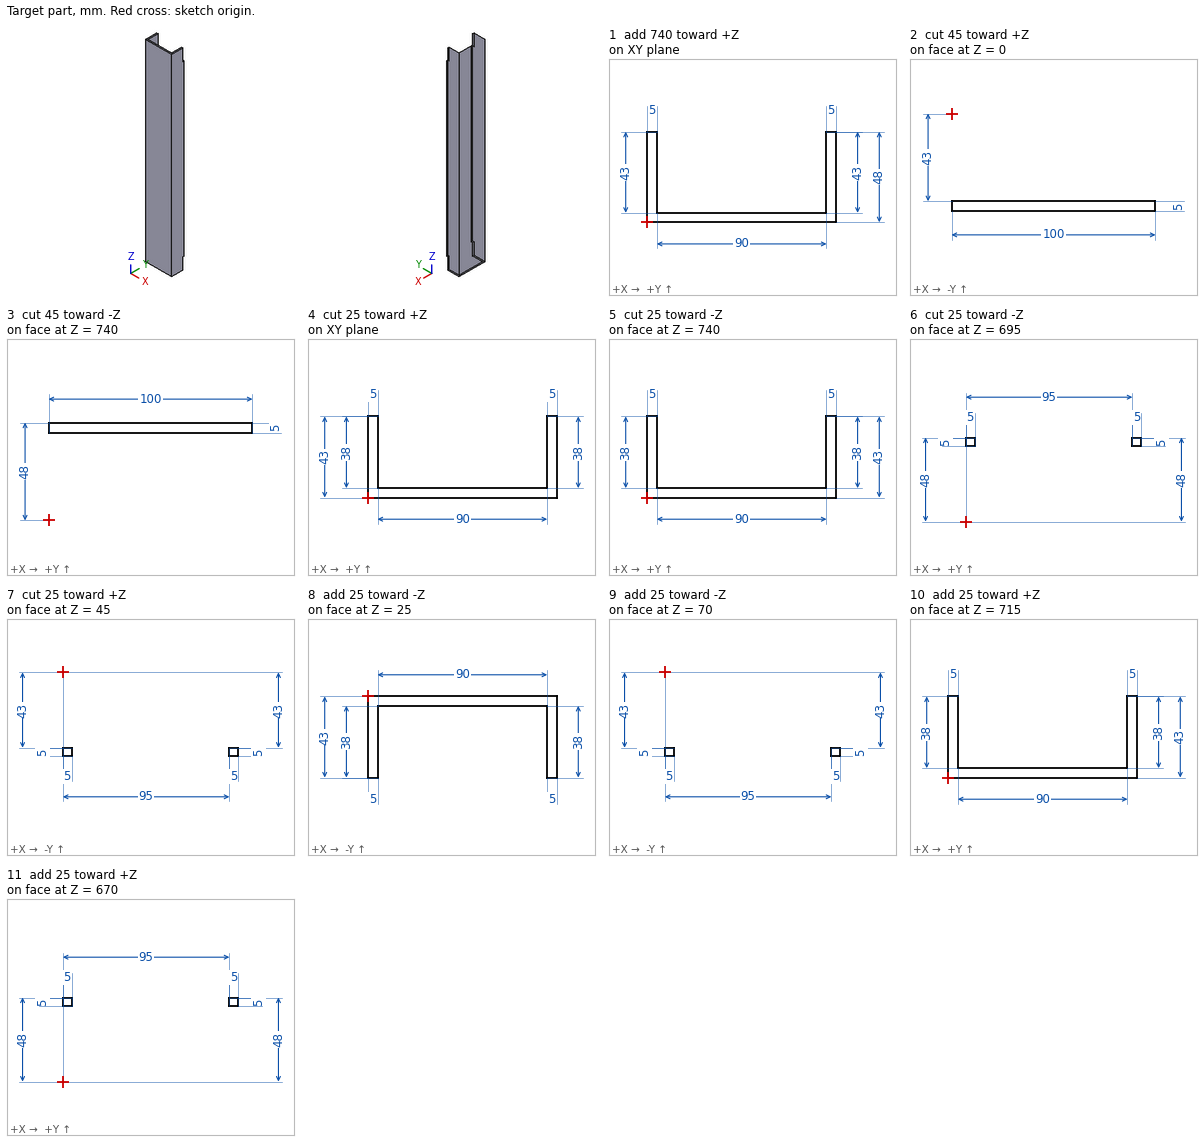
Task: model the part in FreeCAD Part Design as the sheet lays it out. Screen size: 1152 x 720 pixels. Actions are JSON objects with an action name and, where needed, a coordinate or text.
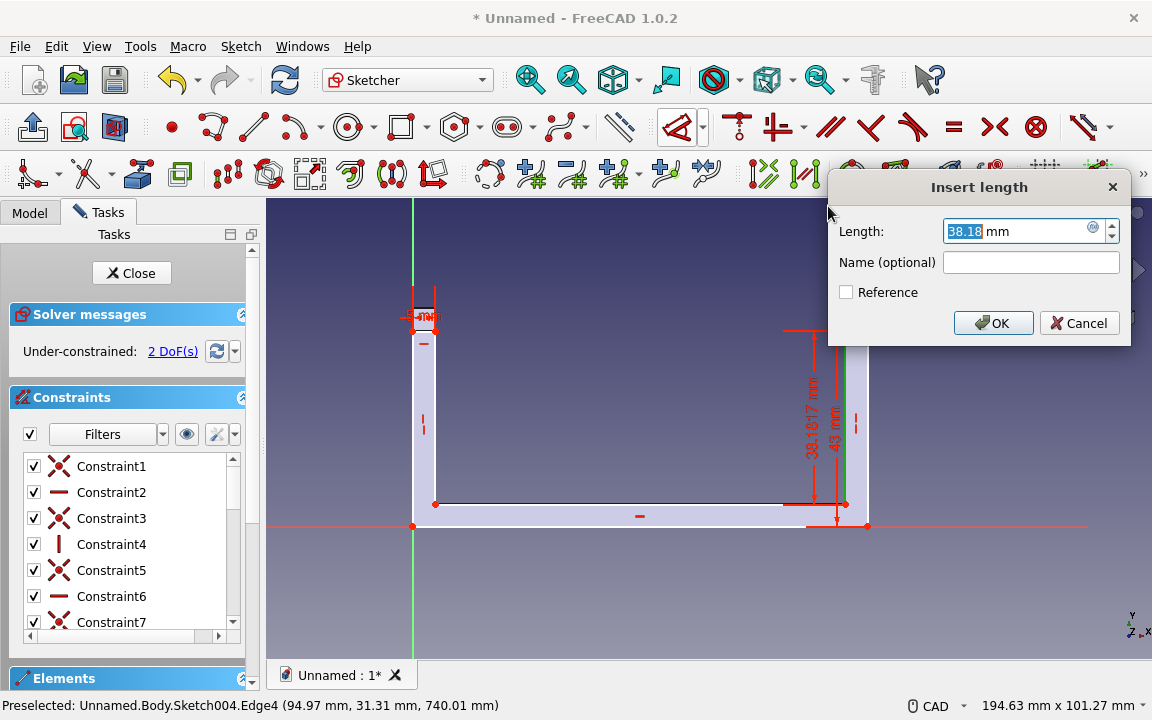
{"action": "type", "text": "38"}
{"action": "key", "text": "Return"}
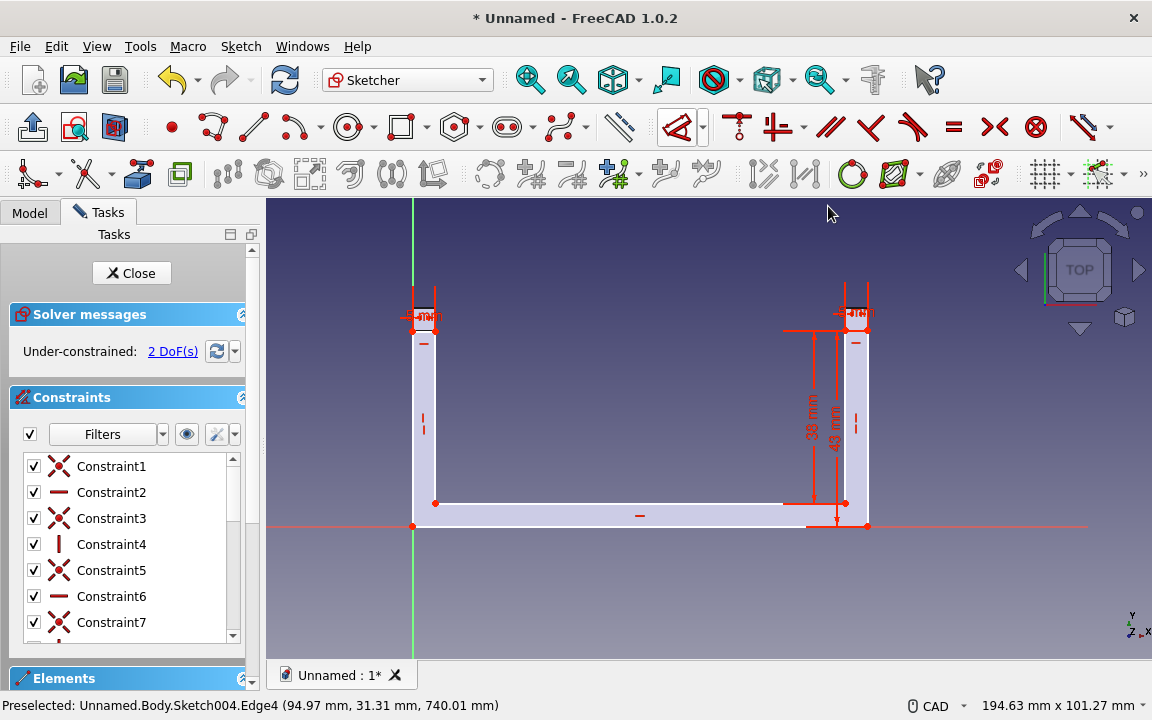
{"action": "left_click", "coordinate": [722, 504]}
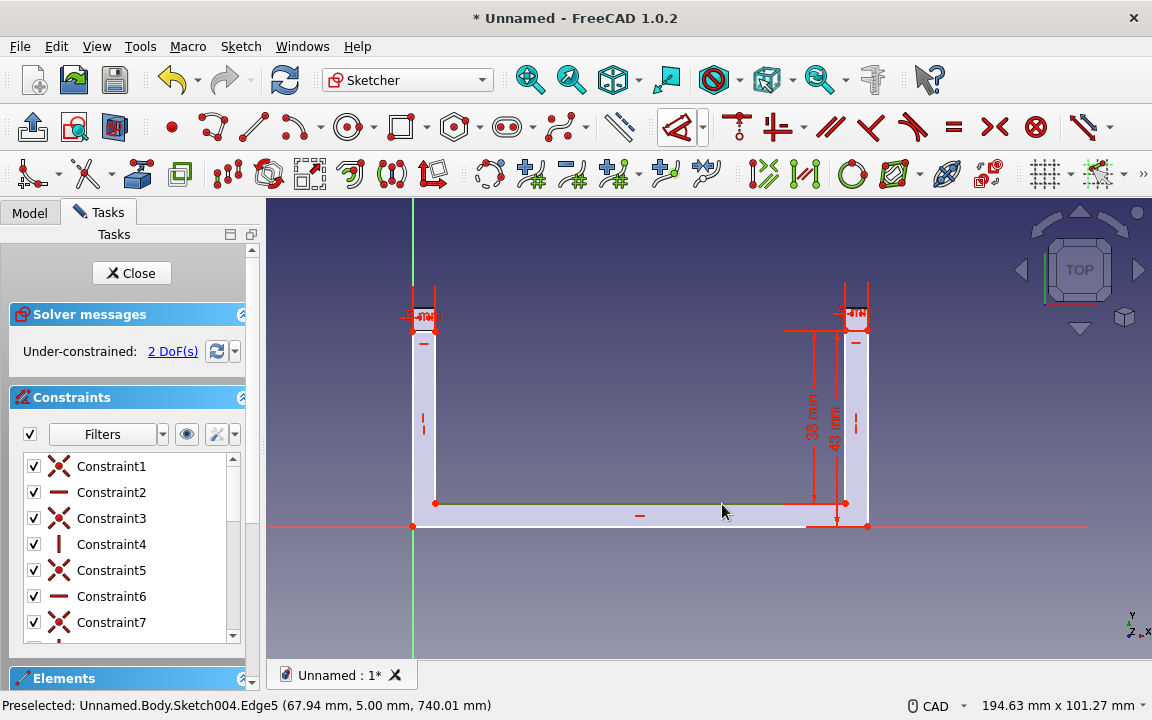
{"action": "key", "text": "l"}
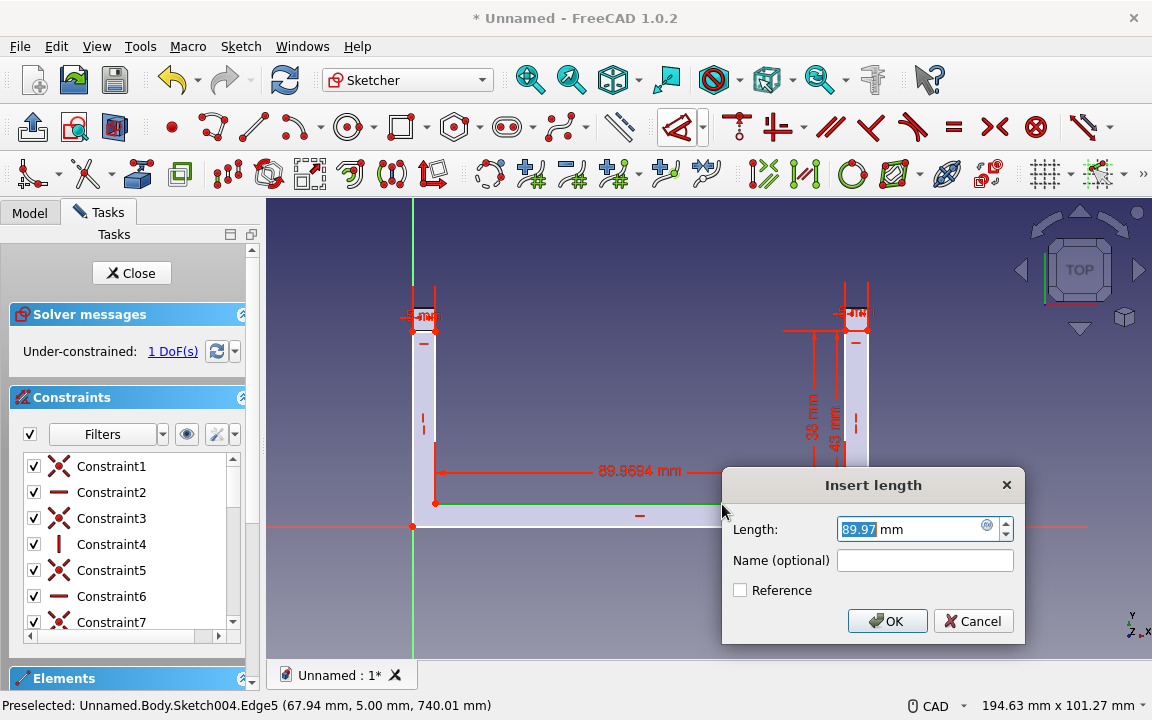
{"action": "type", "text": "90"}
{"action": "key", "text": "Return"}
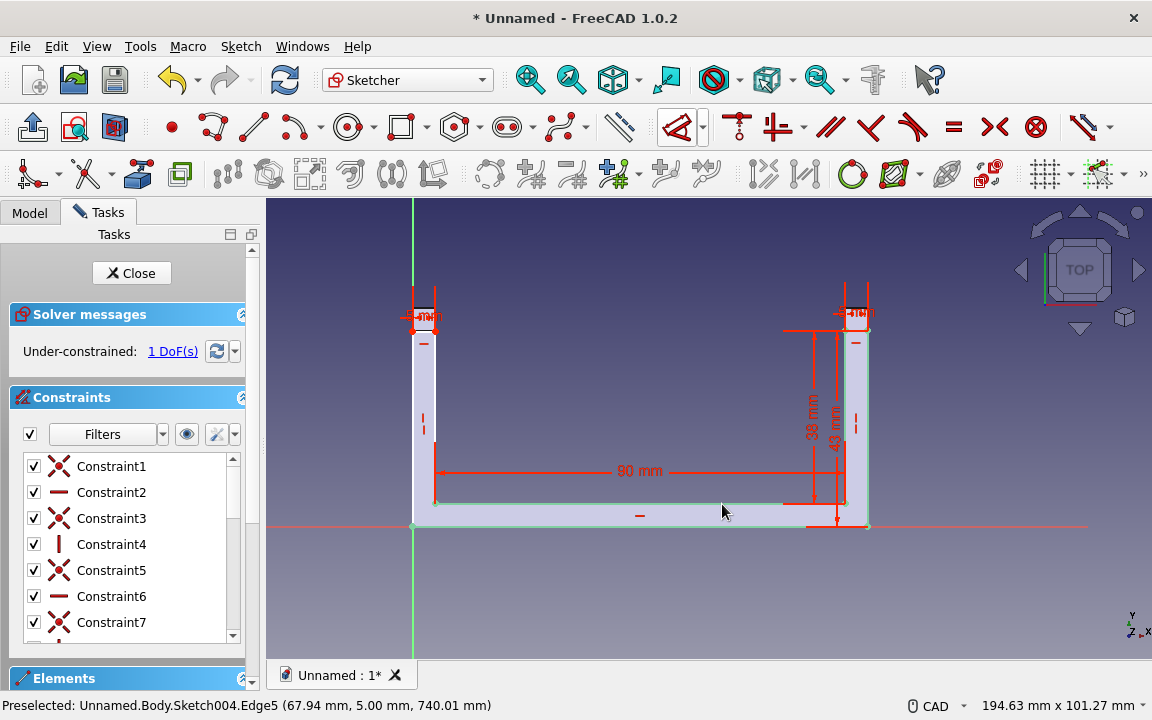
{"action": "left_click", "coordinate": [435, 452]}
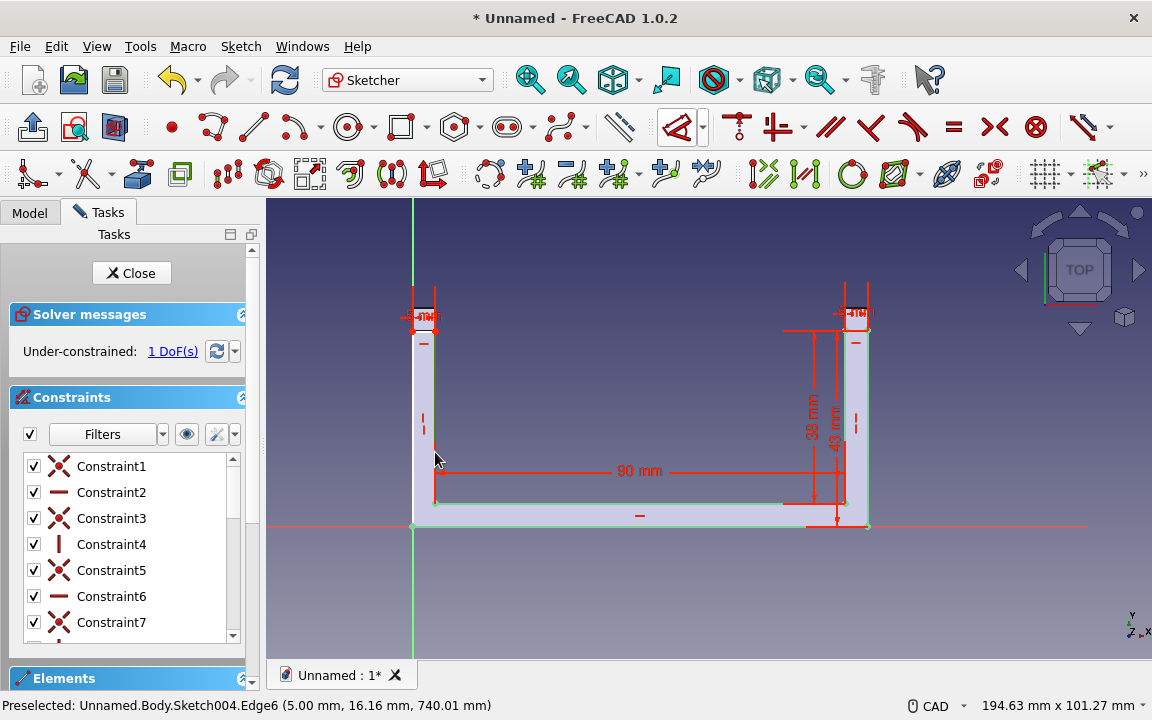
{"action": "key", "text": "i"}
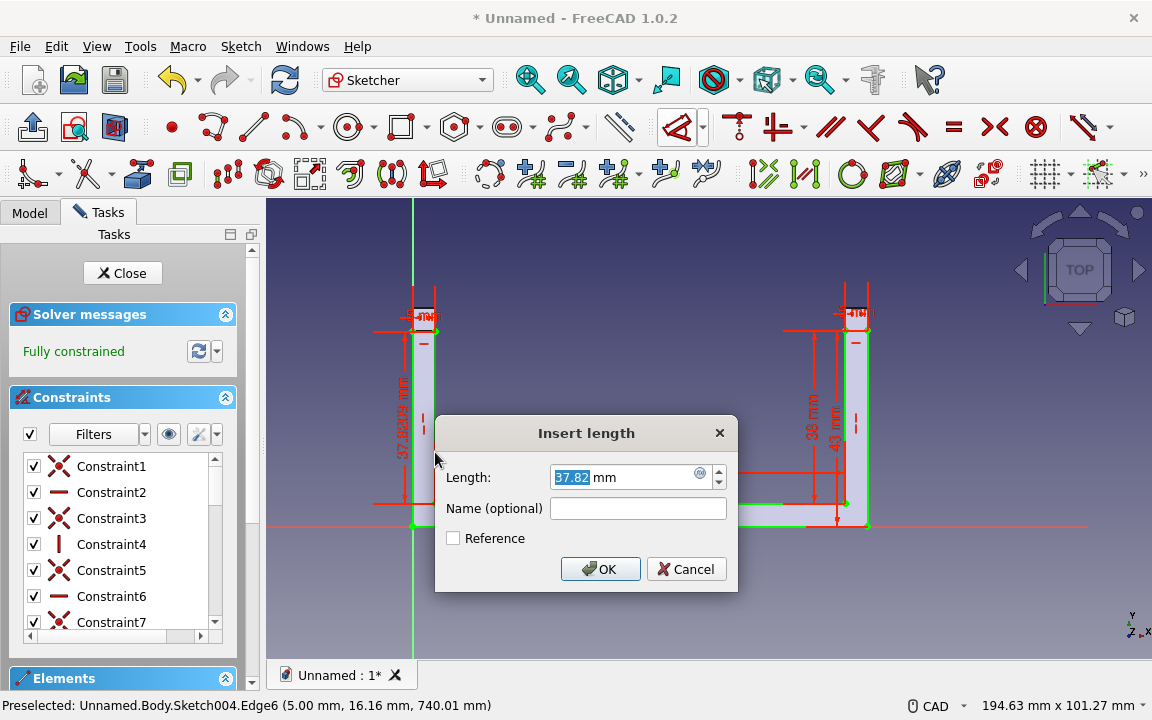
{"action": "type", "text": "38"}
{"action": "key", "text": "Return"}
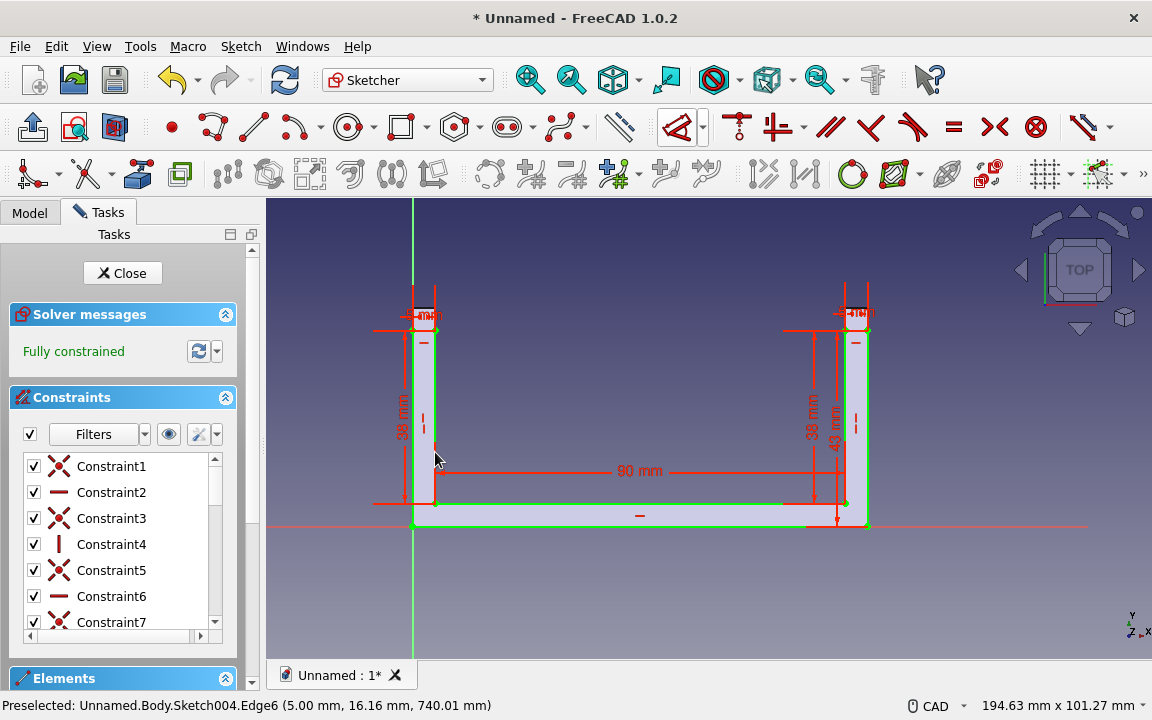
{"action": "left_click", "coordinate": [123, 273]}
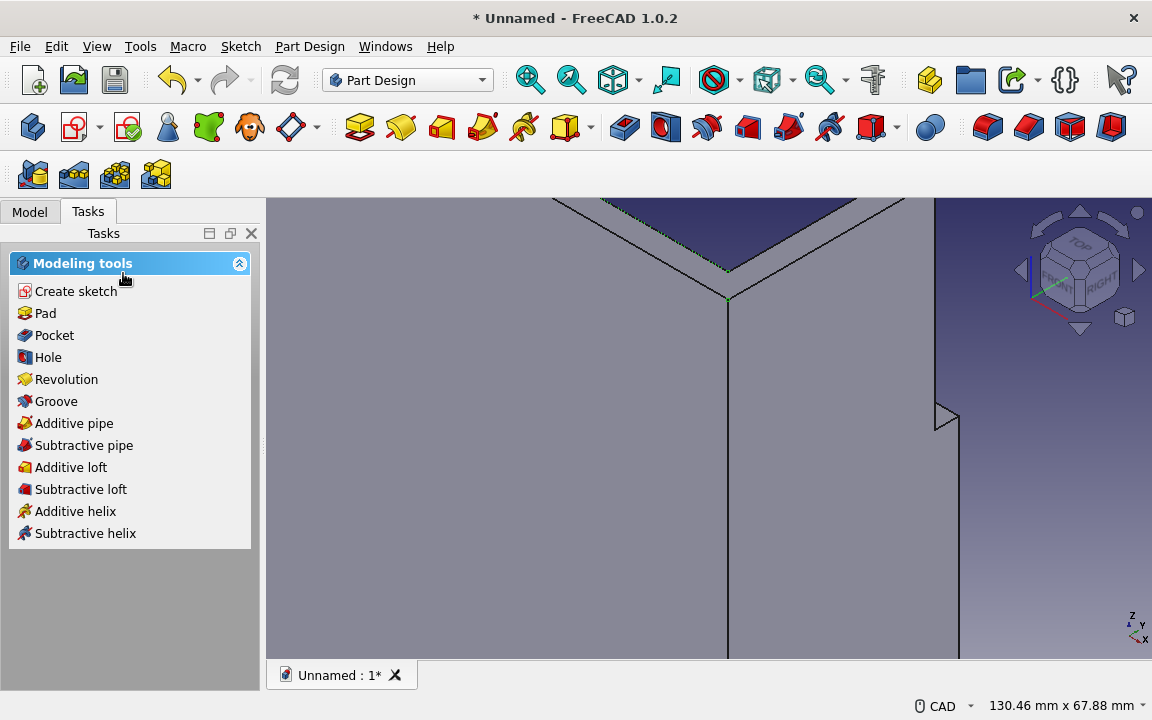
{"action": "left_click", "coordinate": [625, 128]}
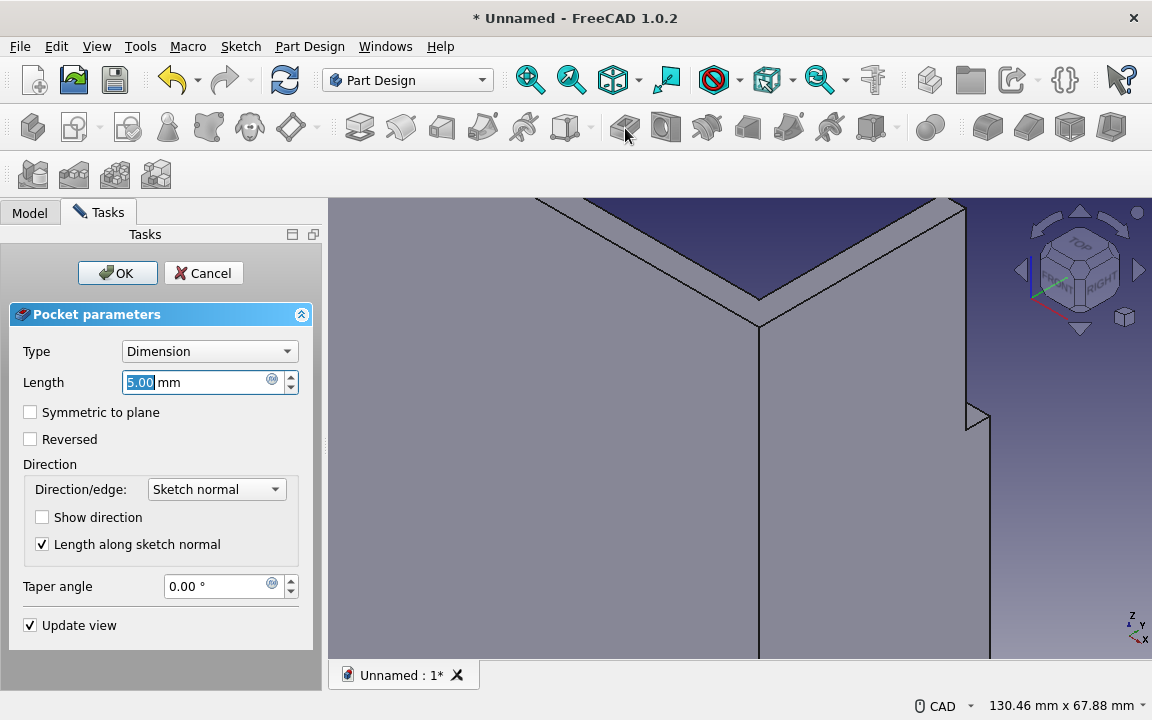
{"action": "type", "text": "25"}
{"action": "key", "text": "Tab"}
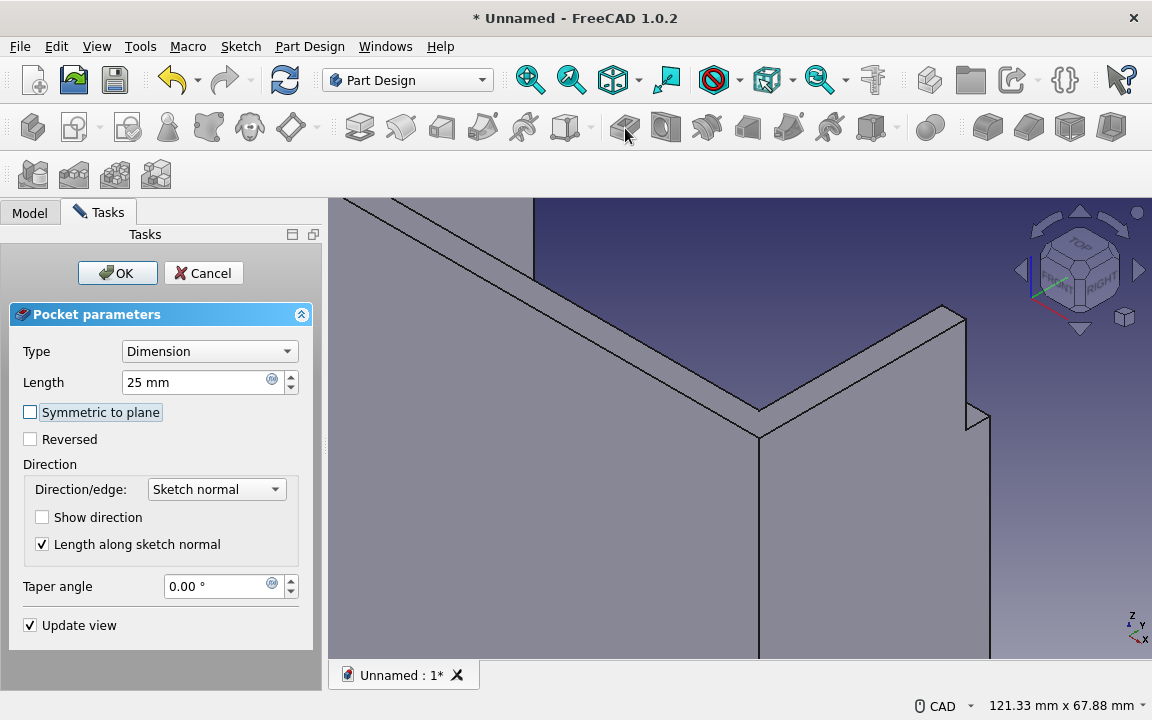
{"action": "left_click", "coordinate": [118, 273]}